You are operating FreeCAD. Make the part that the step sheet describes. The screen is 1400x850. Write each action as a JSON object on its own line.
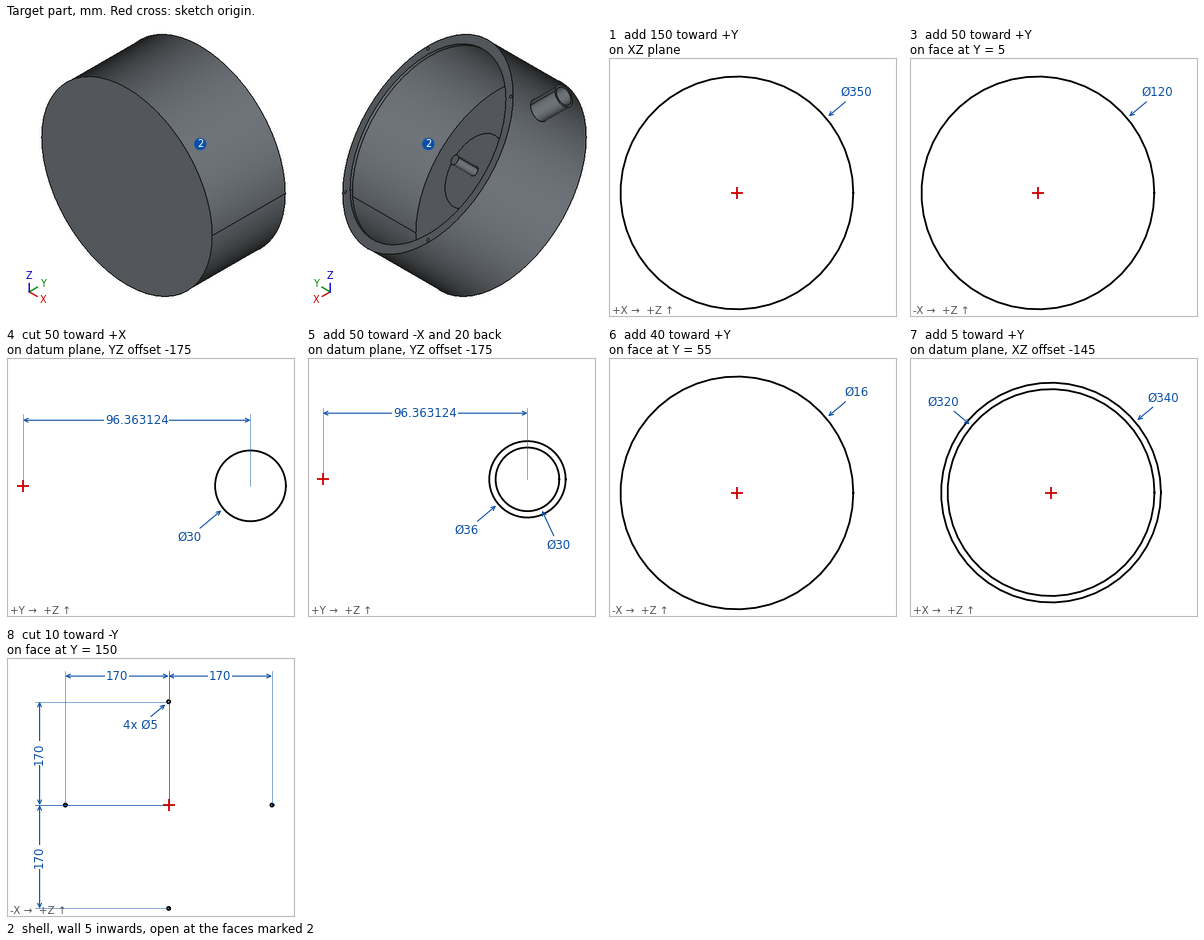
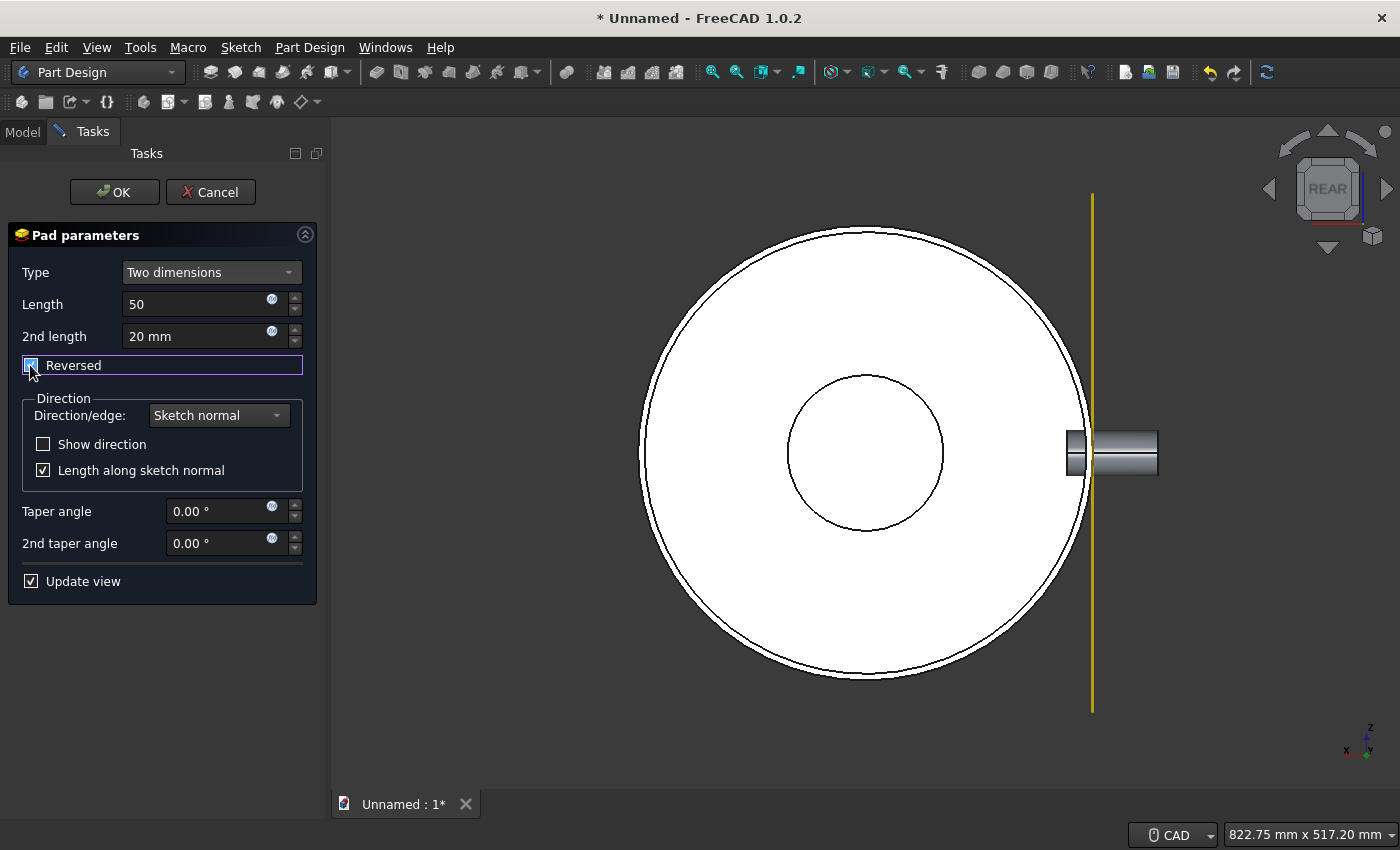
{"action": "left_click", "coordinate": [115, 192]}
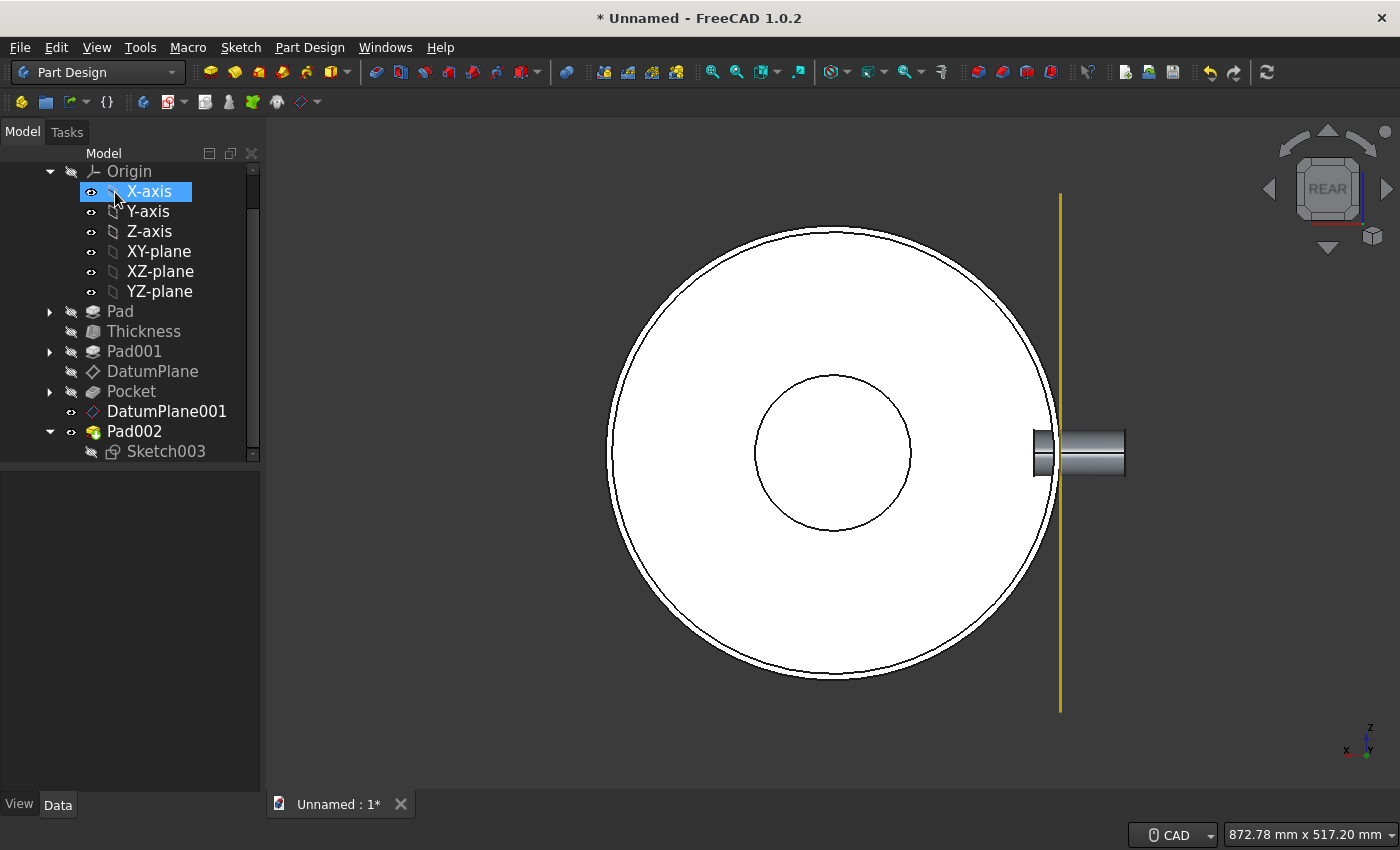
{"action": "left_click", "coordinate": [116, 412]}
{"action": "key", "text": "space"}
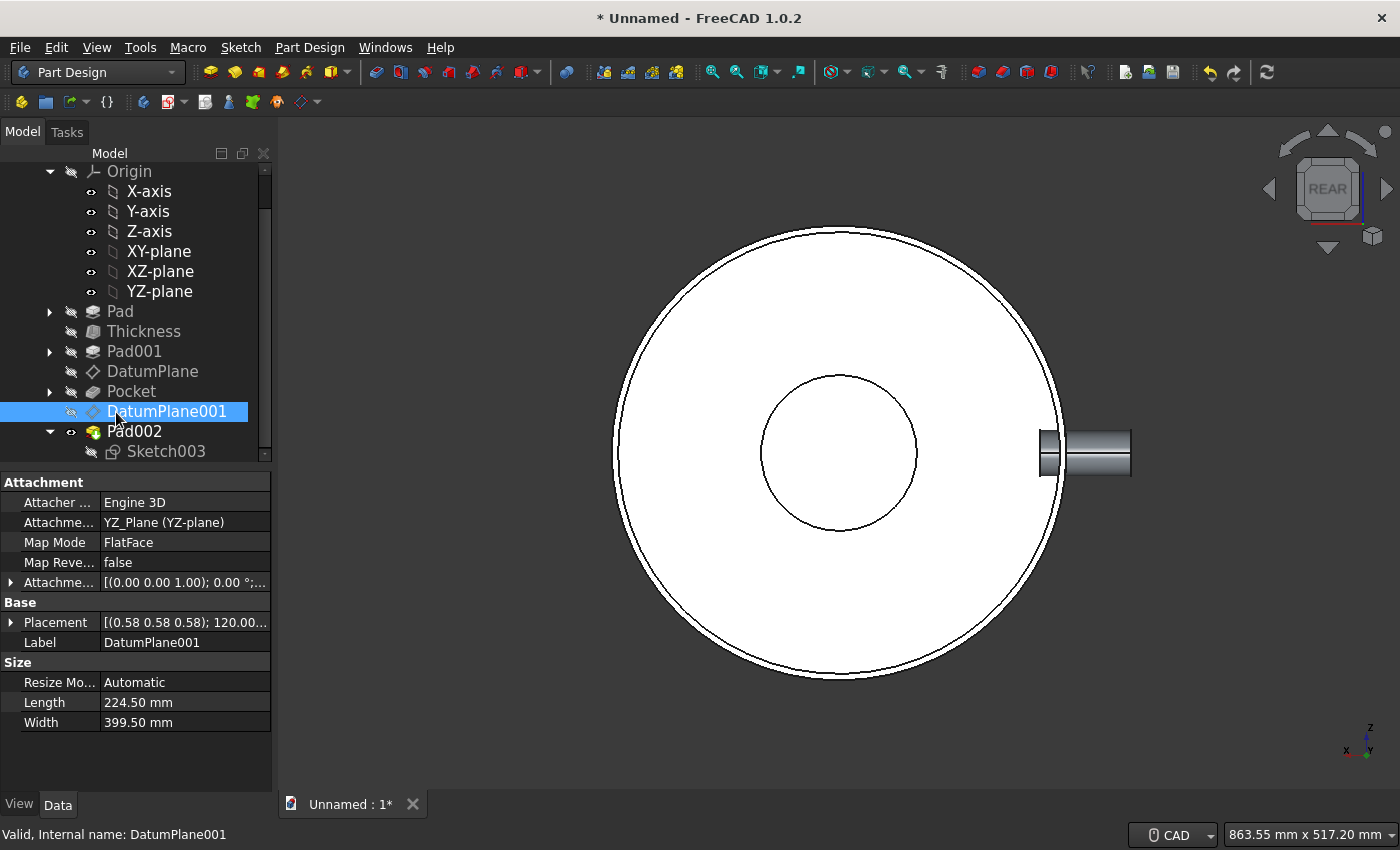
{"action": "left_click", "coordinate": [839, 452]}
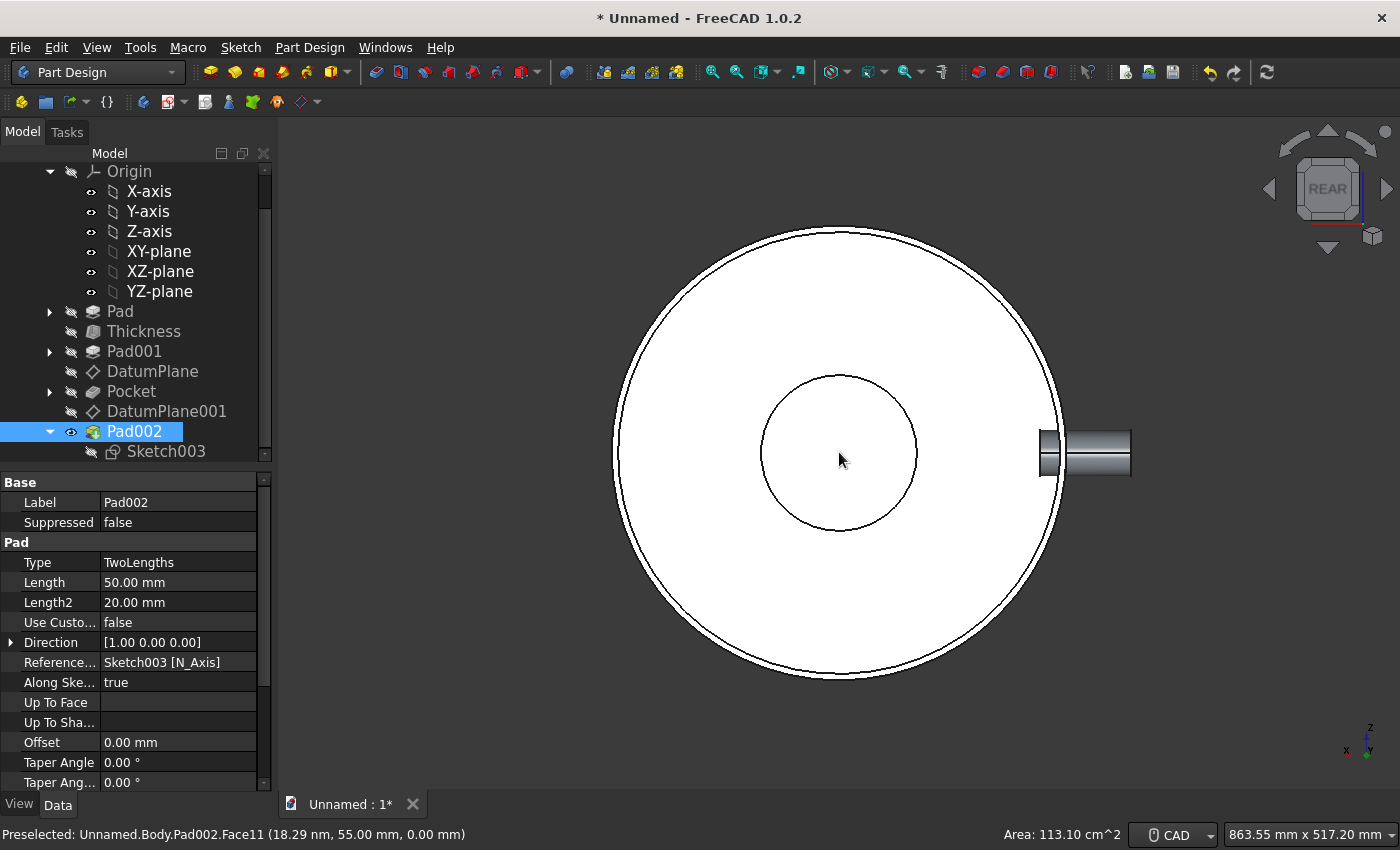
{"action": "left_click", "coordinate": [168, 102]}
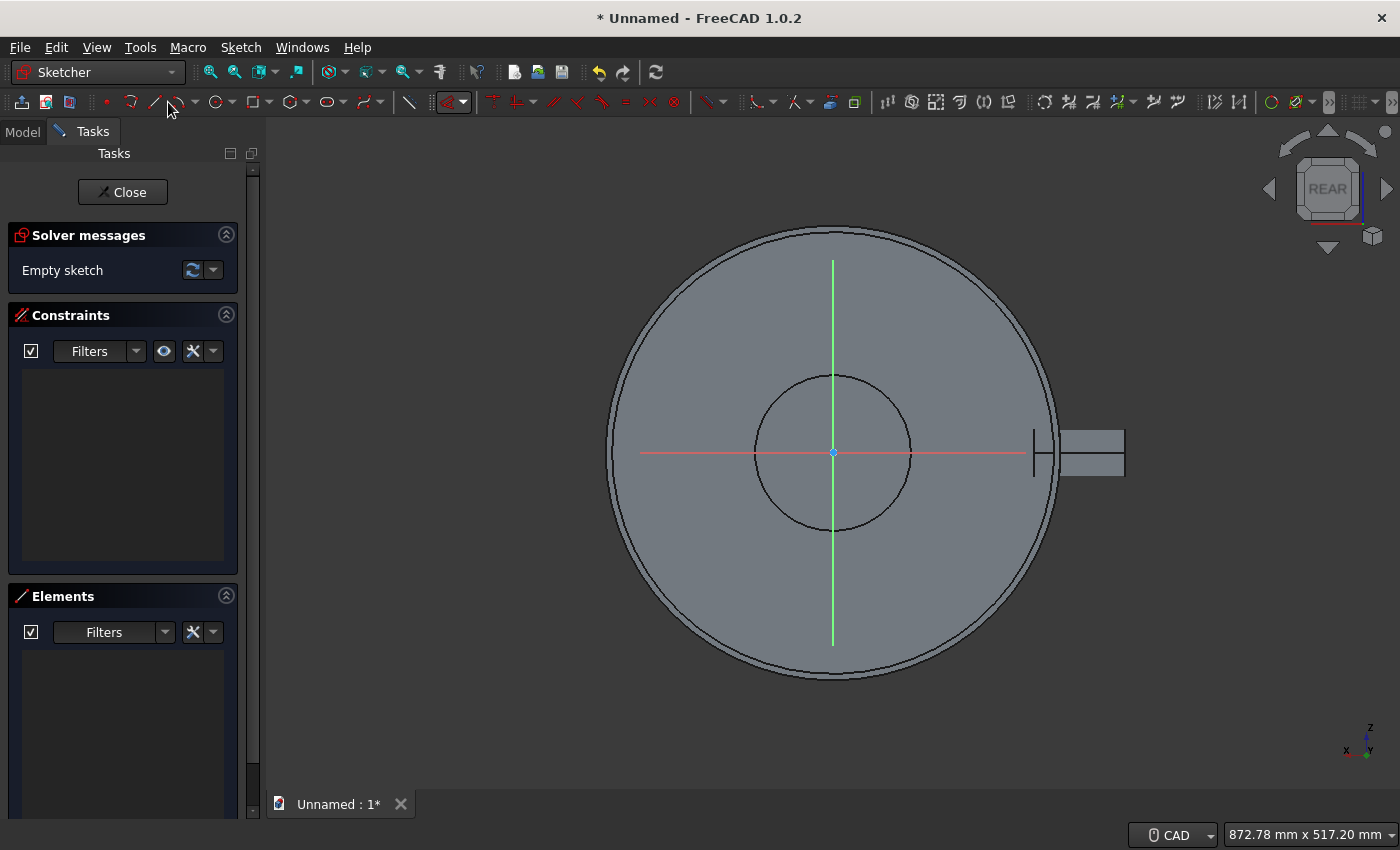
{"action": "left_click", "coordinate": [70, 102]}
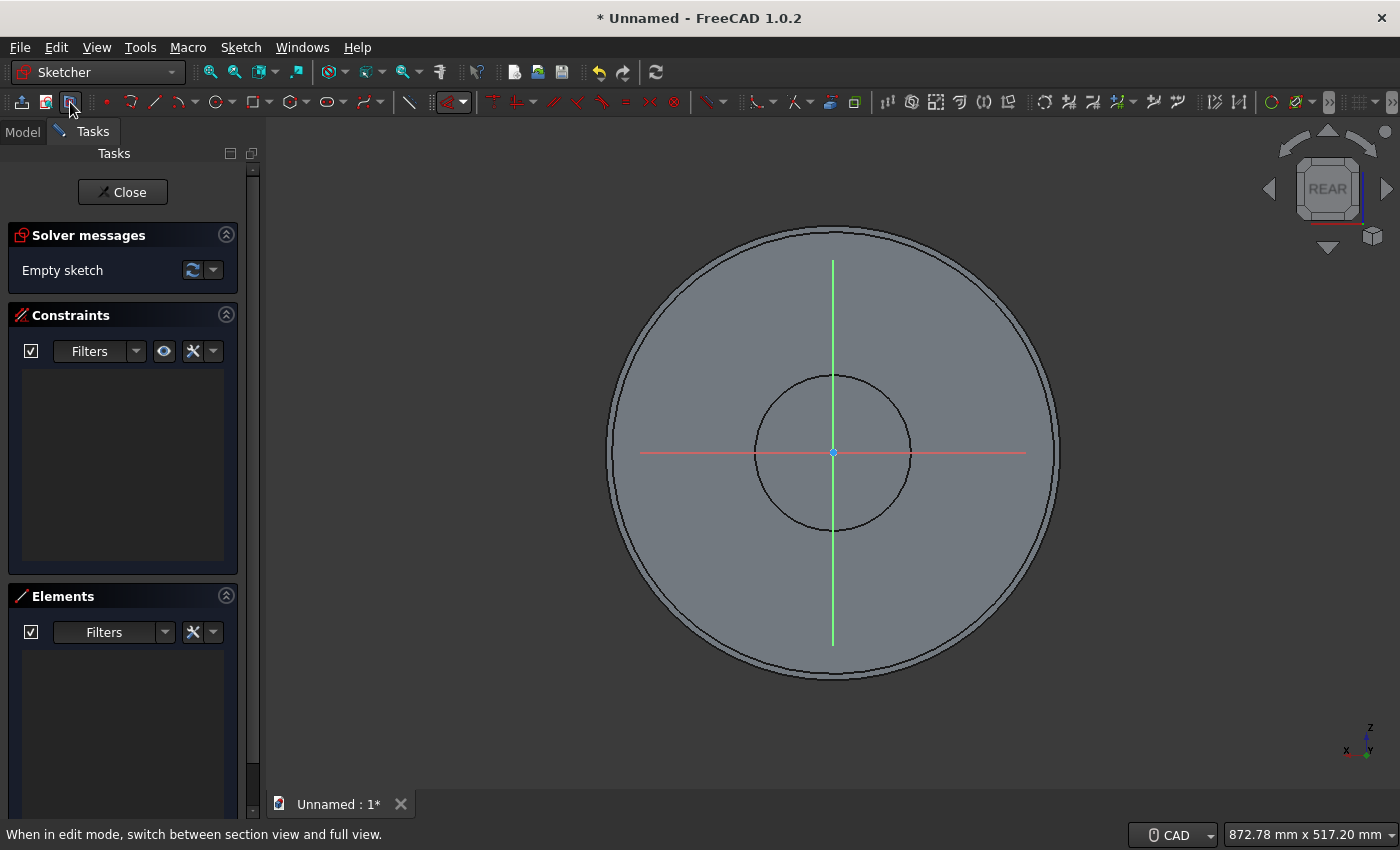
{"action": "scroll", "coordinate": [837, 453], "scroll_direction": "up", "scroll_amount": 15}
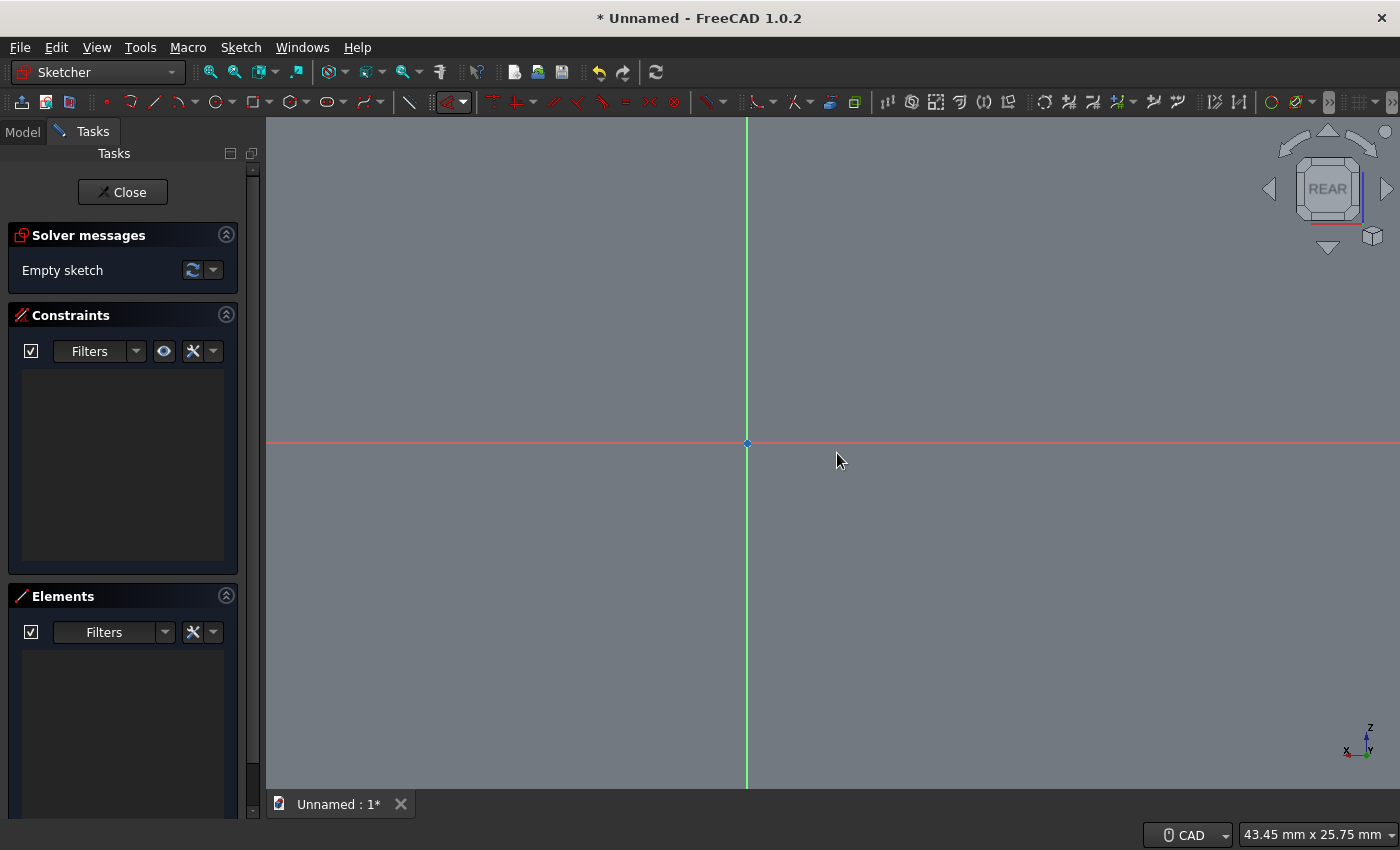
{"action": "left_click", "coordinate": [216, 102]}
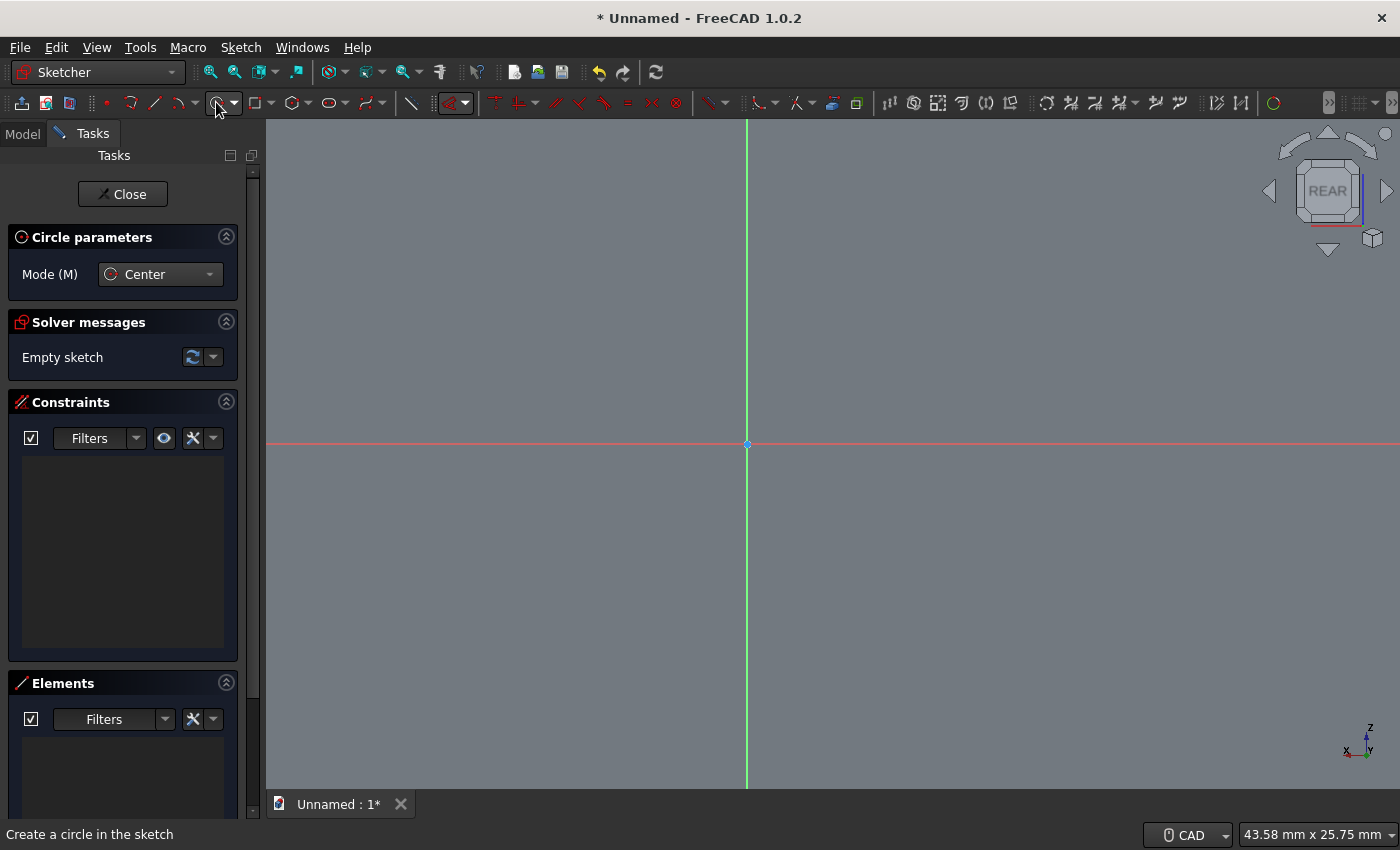
{"action": "left_click", "coordinate": [747, 444]}
{"action": "mouse_move", "coordinate": [894, 297]}